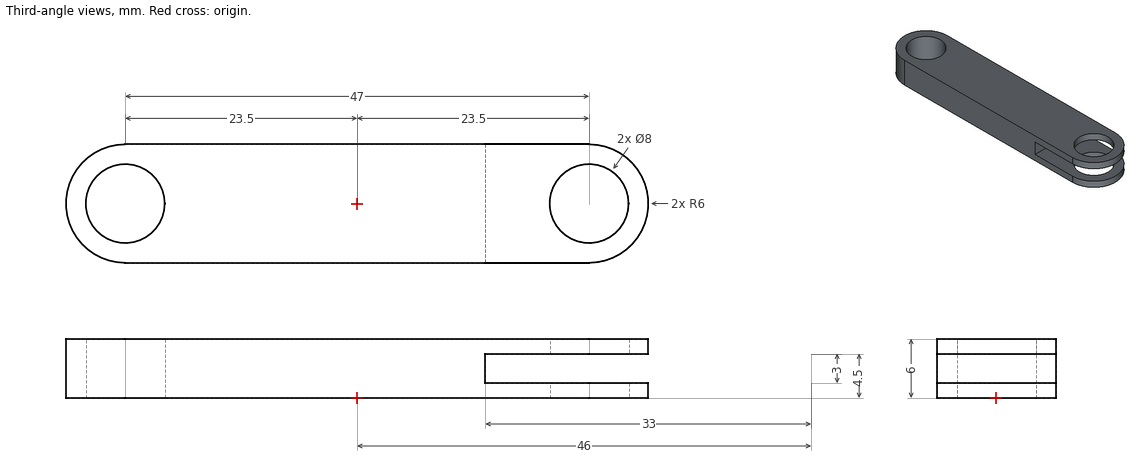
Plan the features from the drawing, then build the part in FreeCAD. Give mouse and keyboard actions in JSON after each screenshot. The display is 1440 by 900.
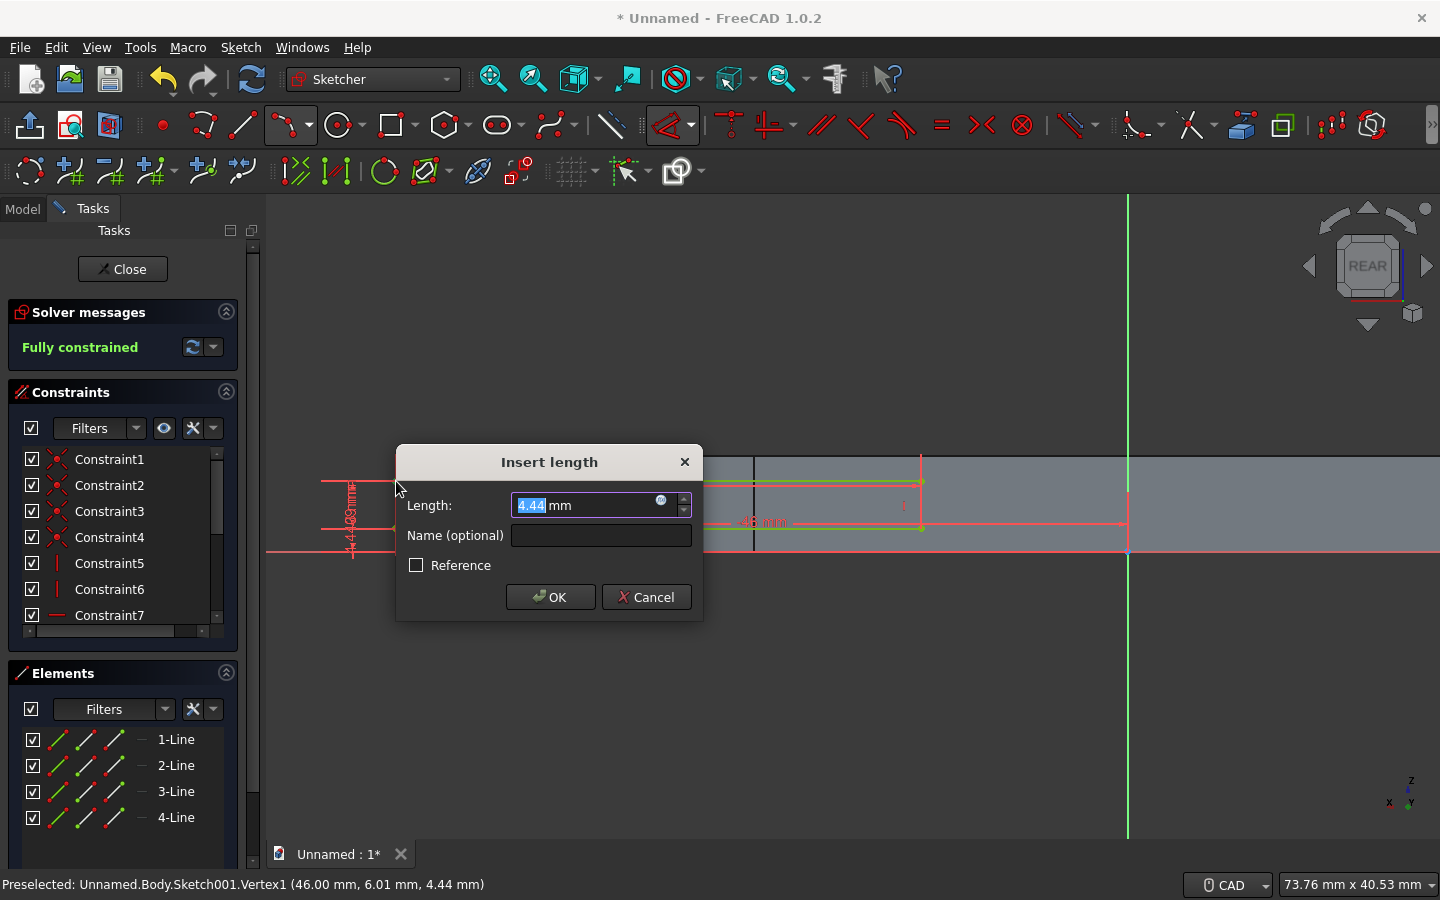
{"action": "type", "text": "4.5"}
{"action": "key", "text": "Return"}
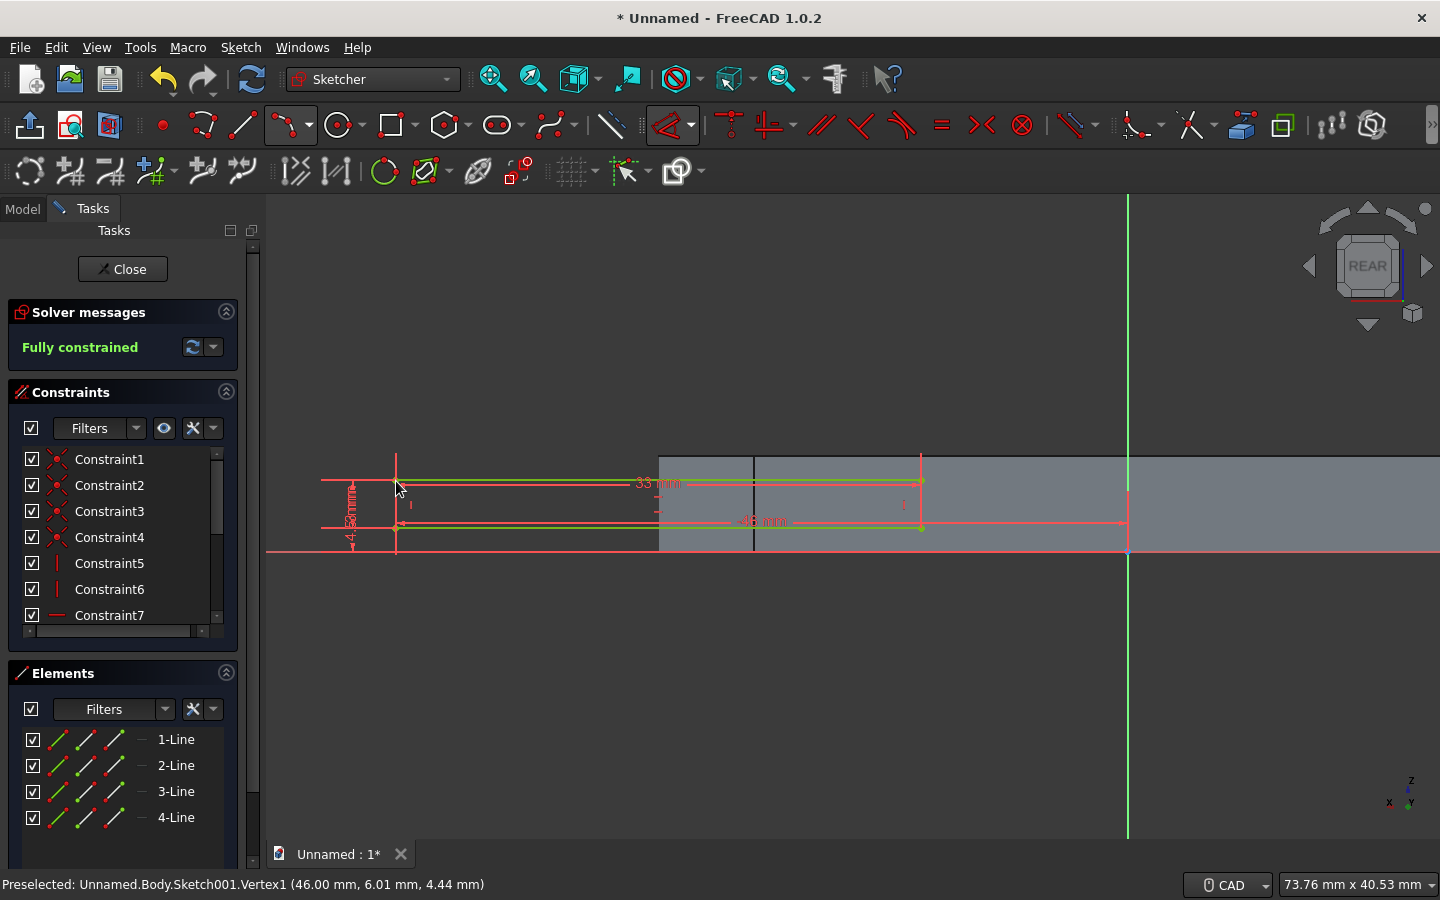
{"action": "left_click", "coordinate": [123, 269]}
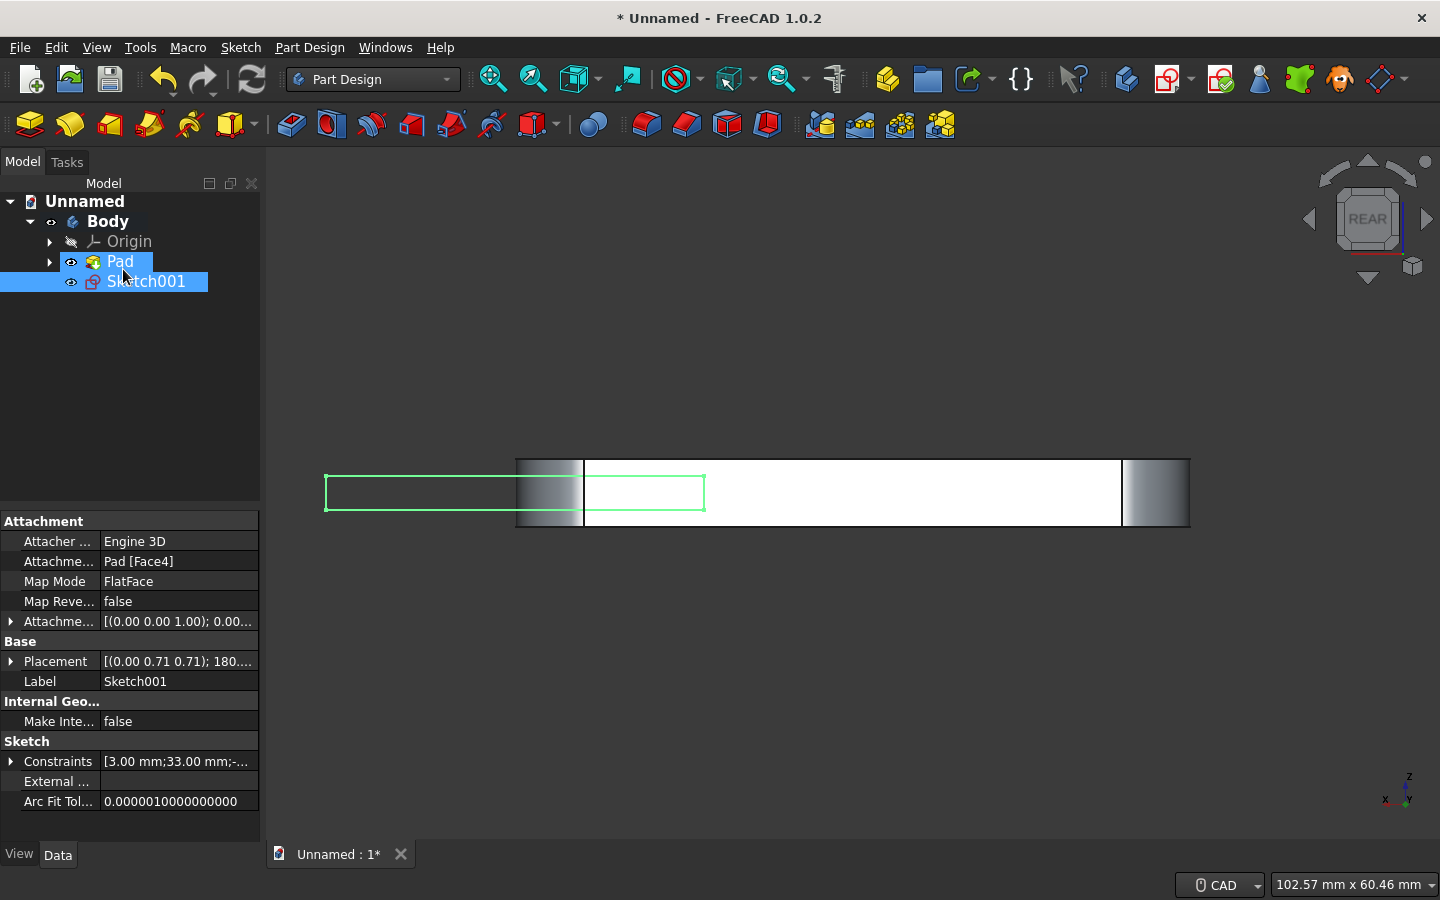
{"action": "left_click", "coordinate": [292, 124]}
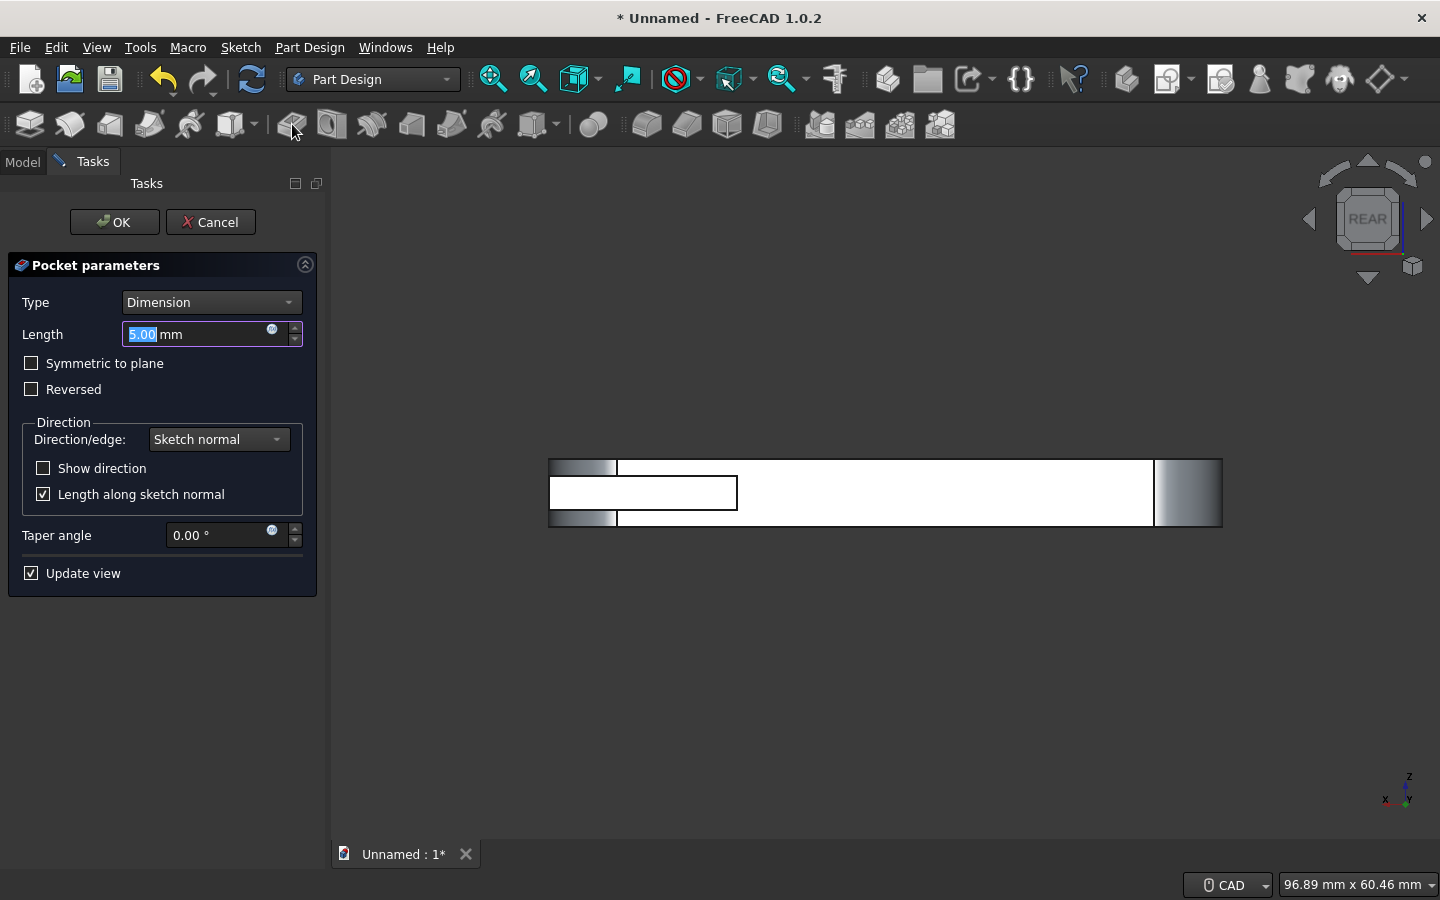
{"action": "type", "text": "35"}
{"action": "key", "text": "Tab"}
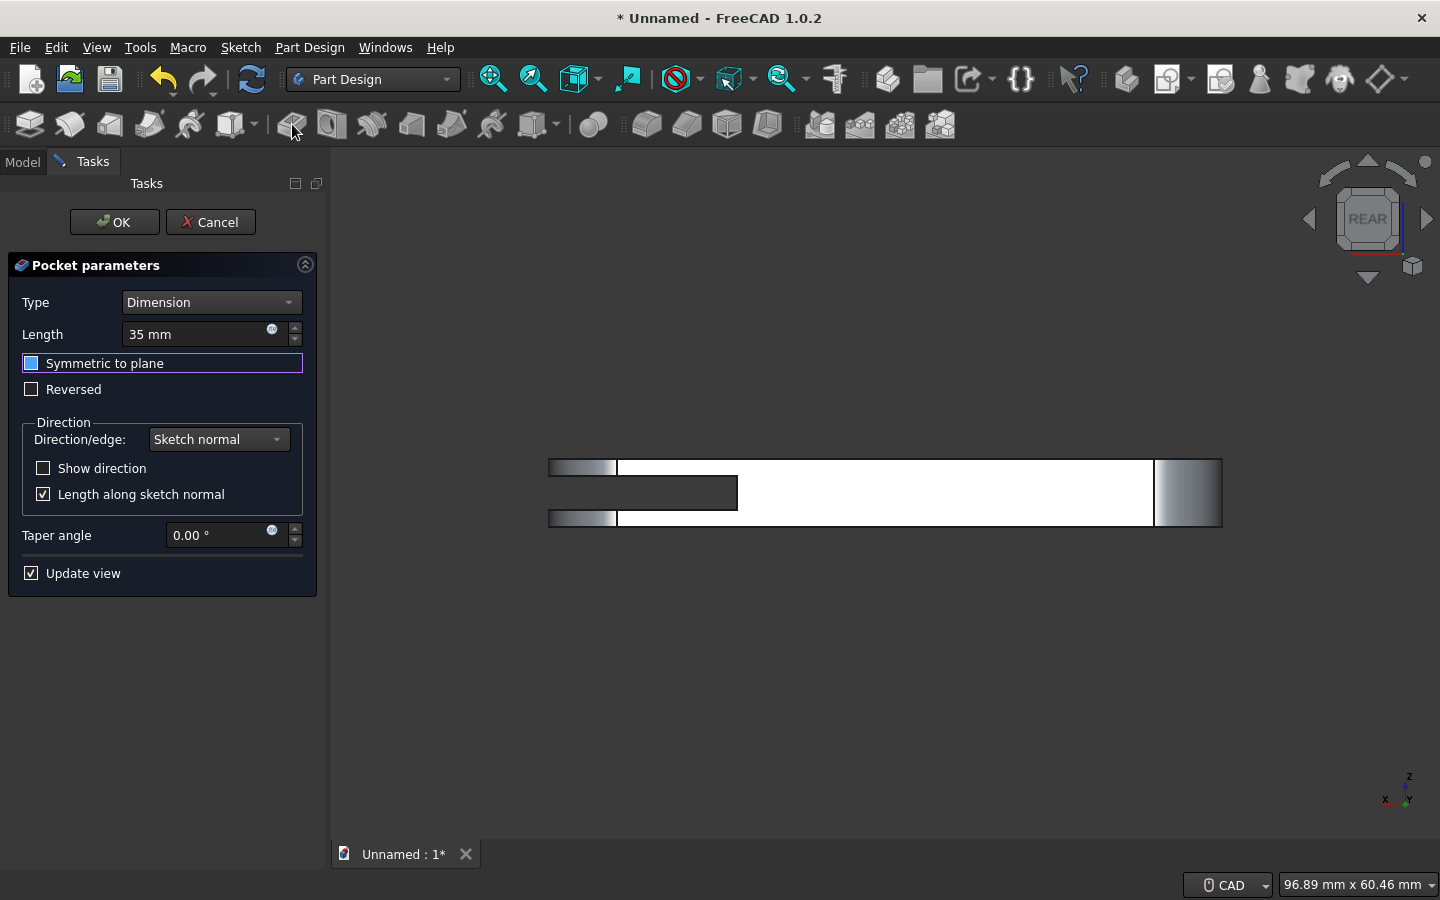
{"action": "left_click", "coordinate": [115, 222]}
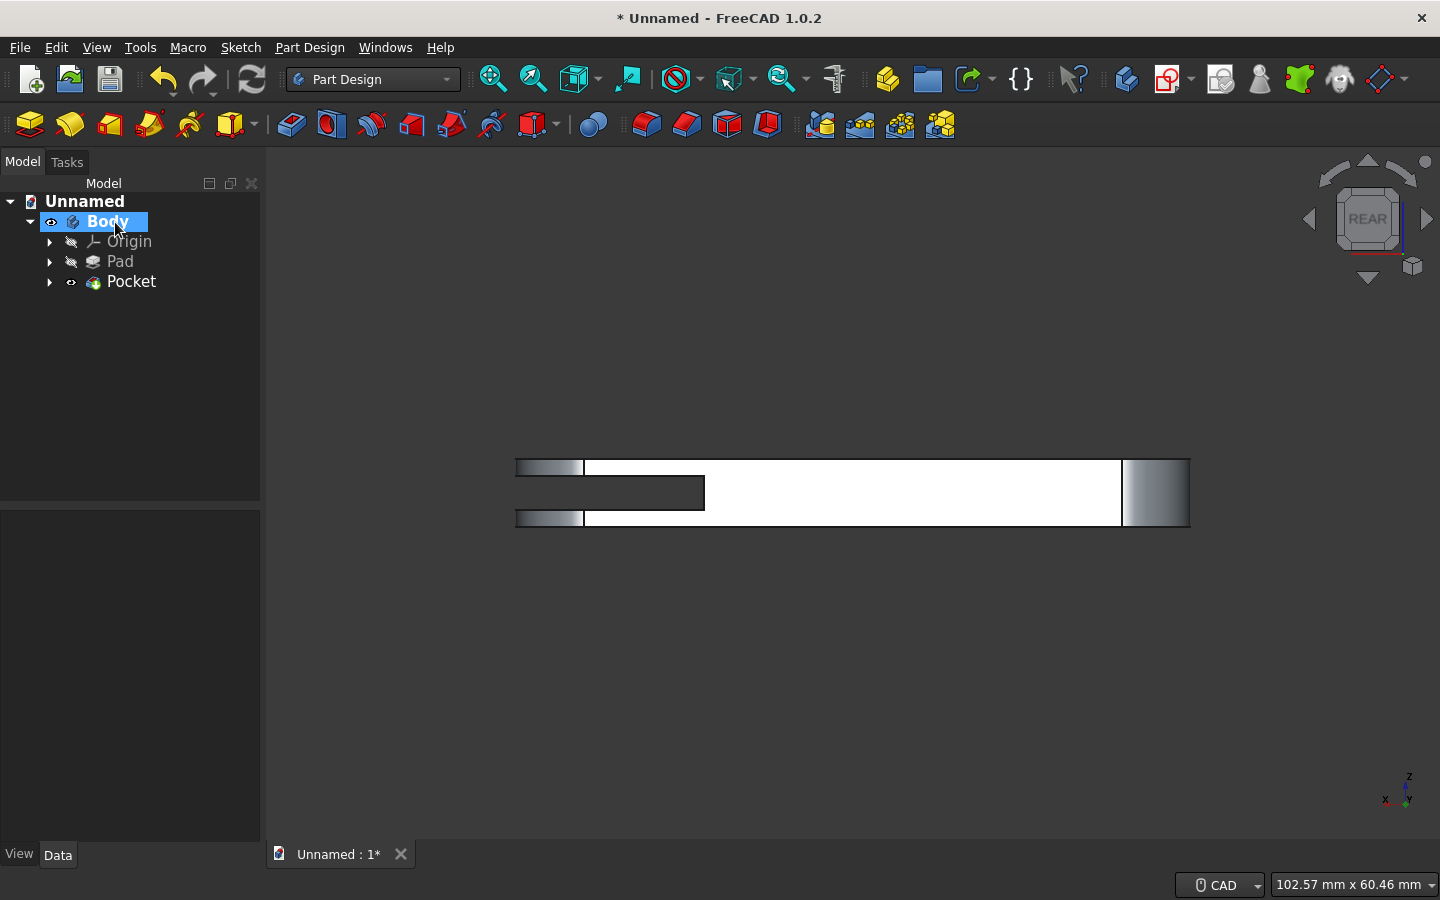
{"action": "key", "text": "0"}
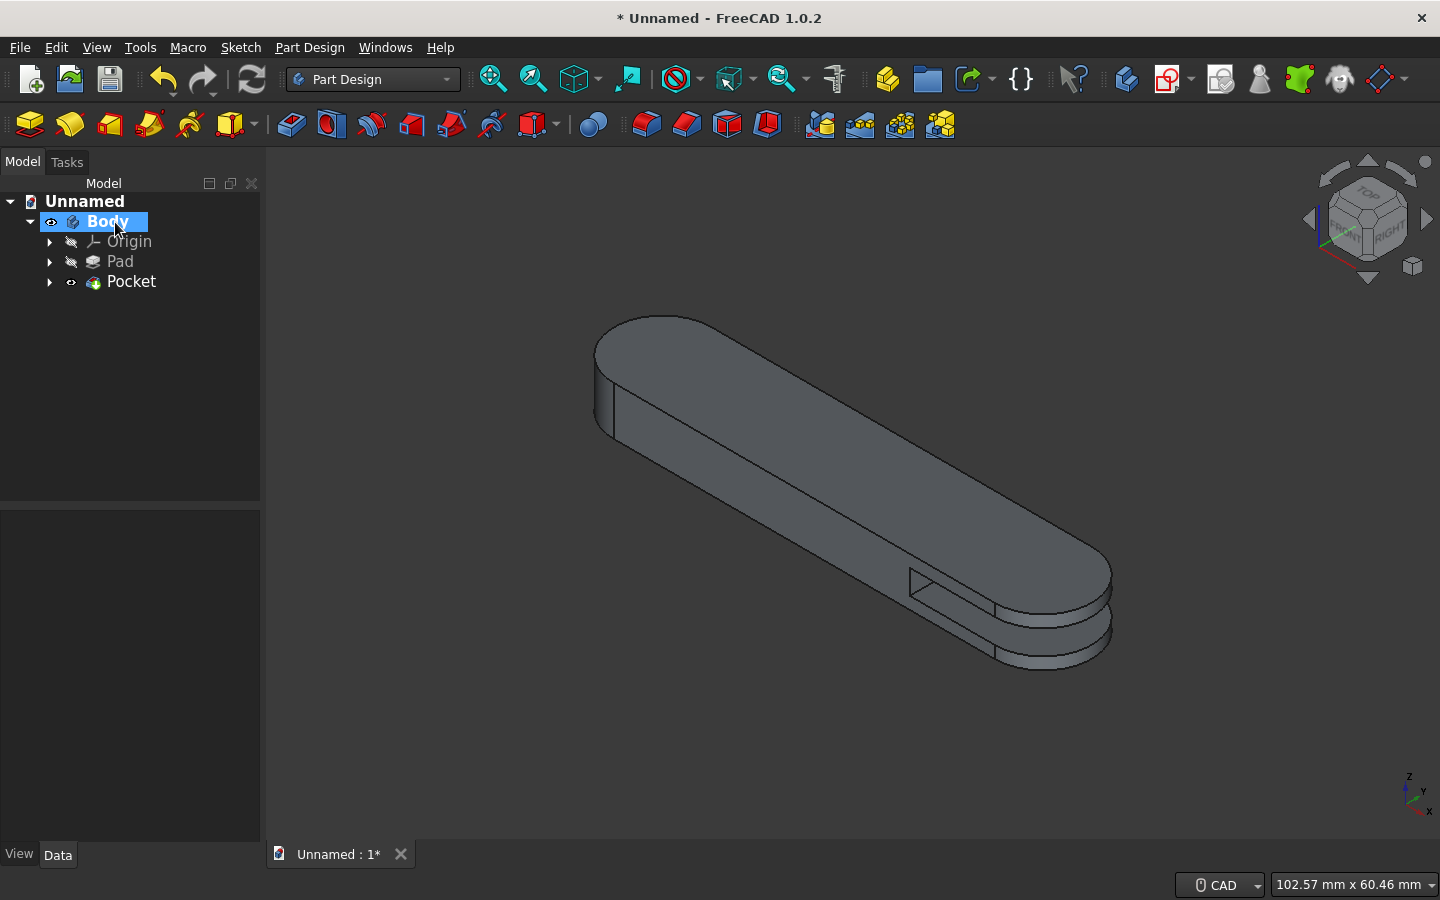
{"action": "left_click", "coordinate": [989, 543]}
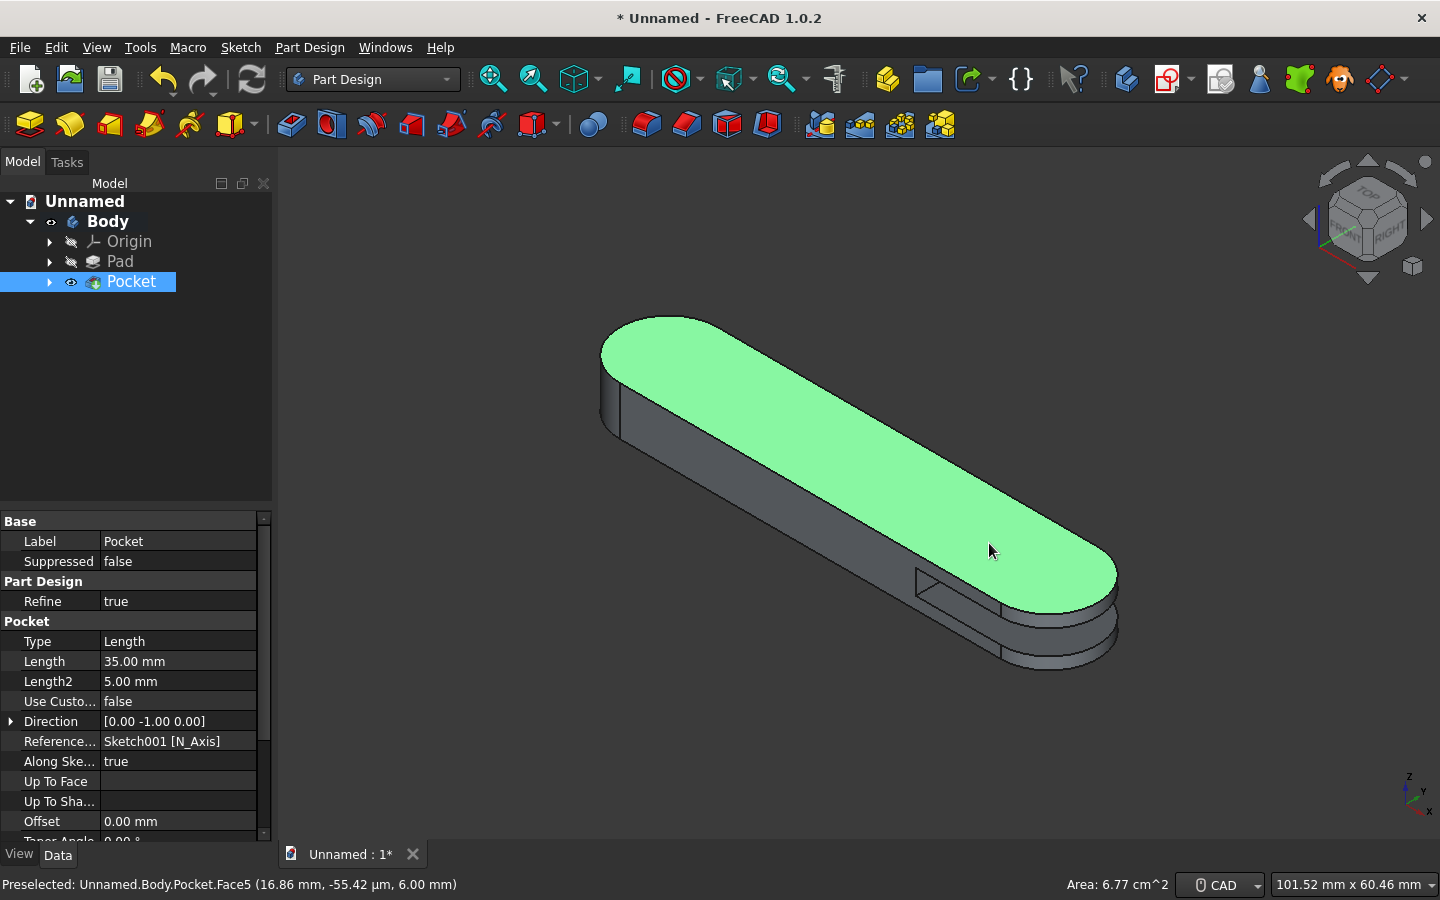
{"action": "left_click", "coordinate": [1168, 80]}